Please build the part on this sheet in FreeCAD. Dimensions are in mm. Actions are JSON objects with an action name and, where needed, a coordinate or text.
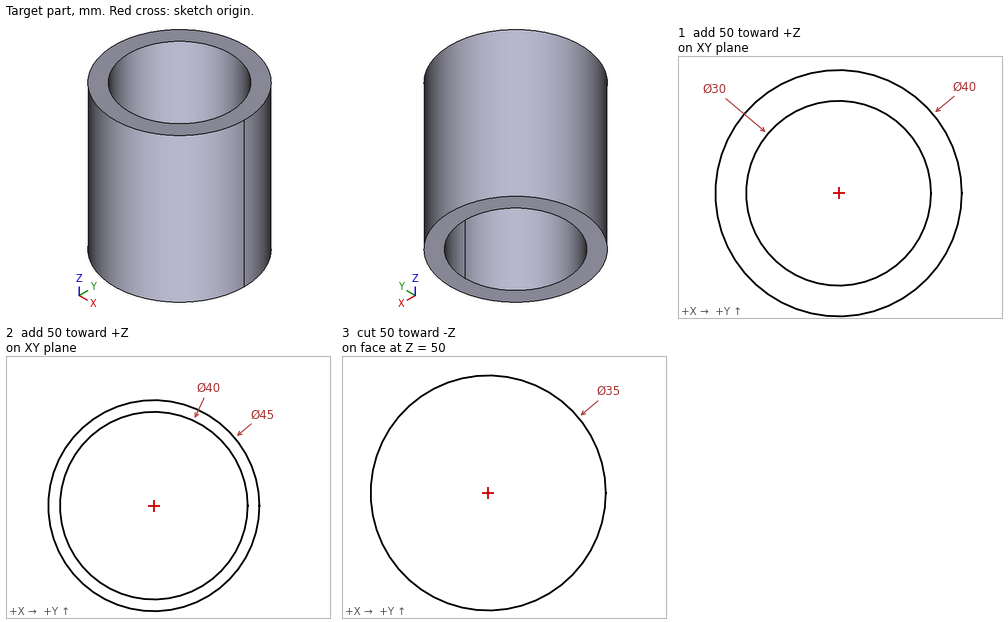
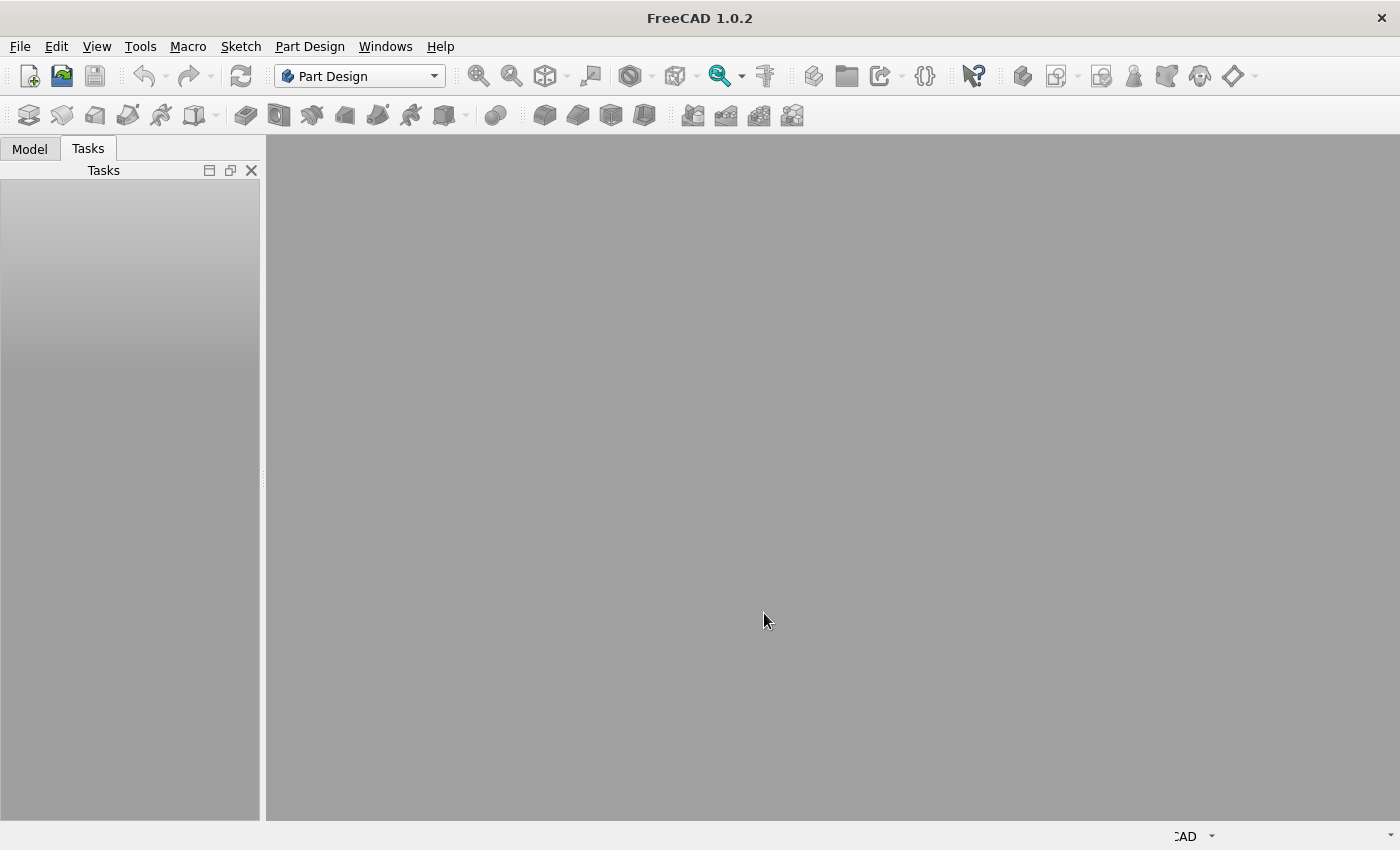
{"action": "left_click", "coordinate": [29, 76]}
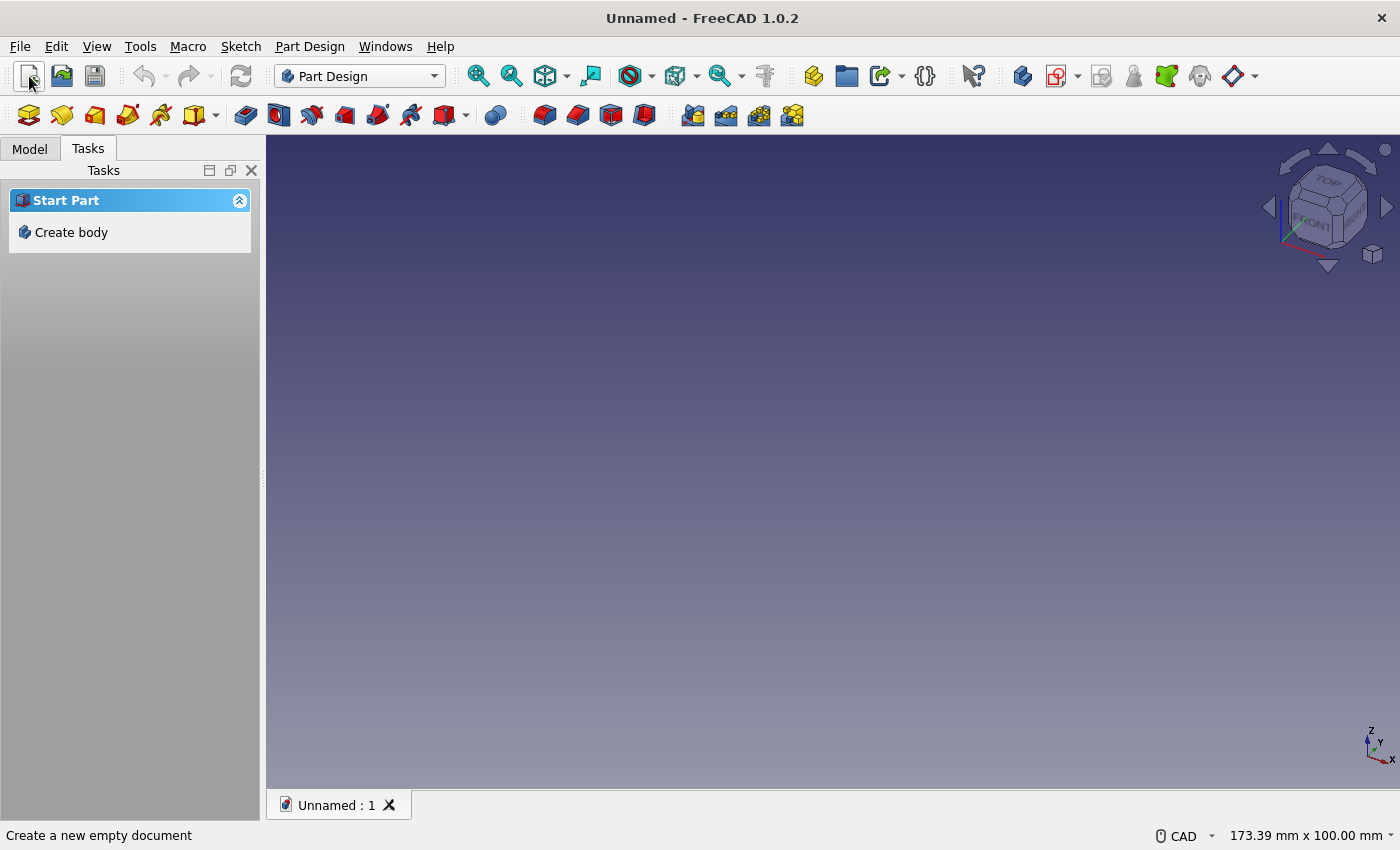
{"action": "left_click", "coordinate": [1056, 76]}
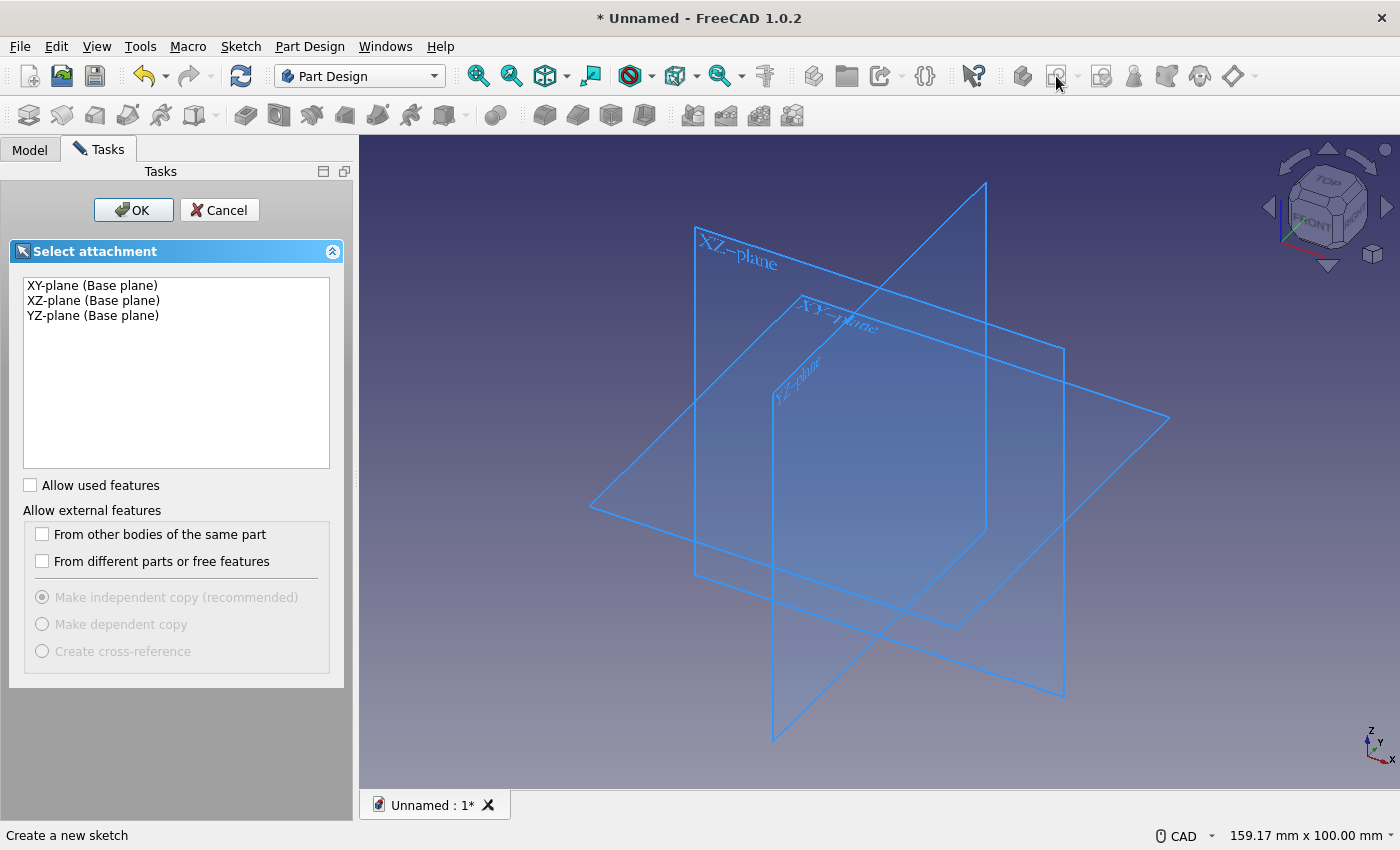
{"action": "left_click", "coordinate": [84, 286]}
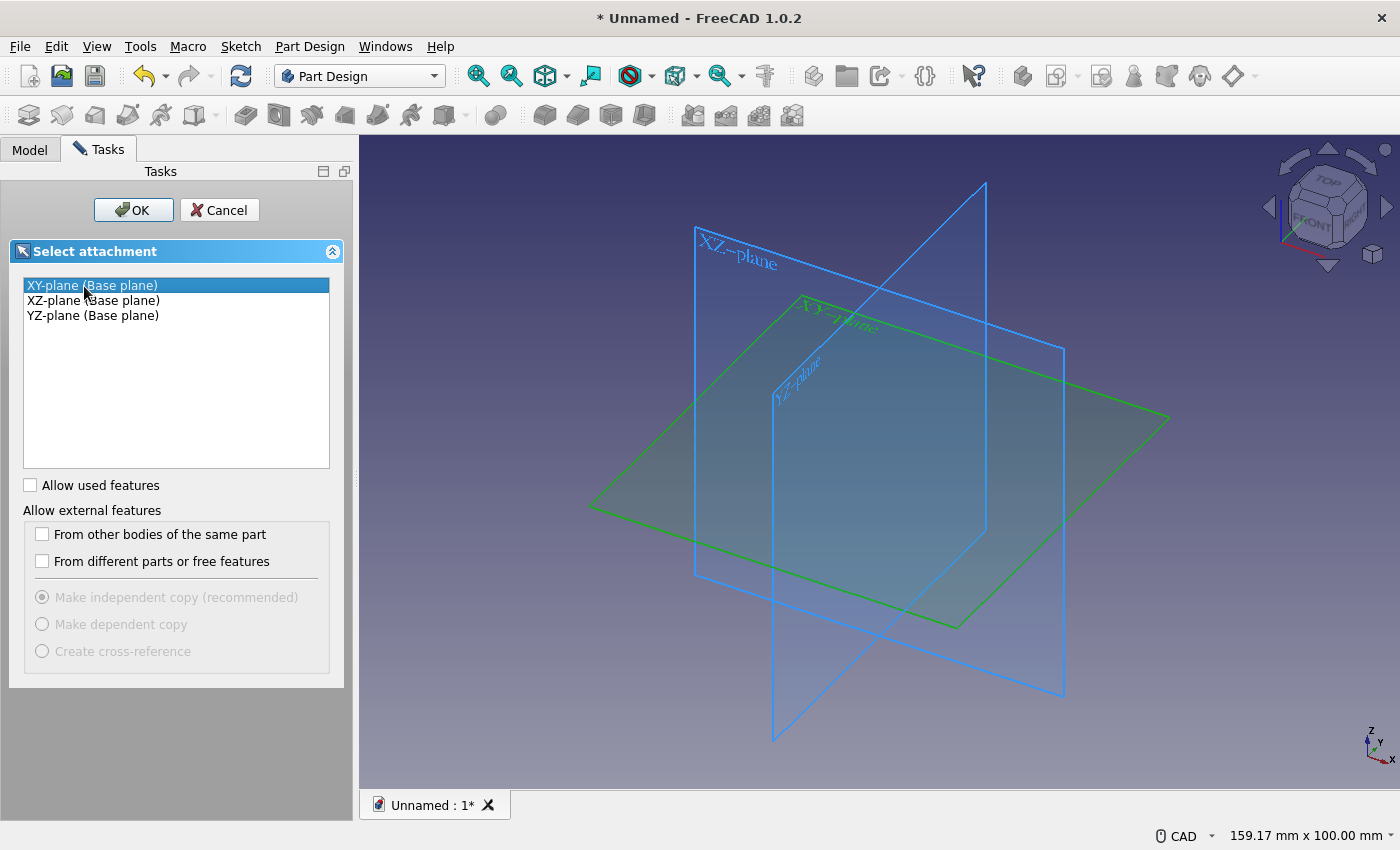
{"action": "left_click", "coordinate": [134, 210]}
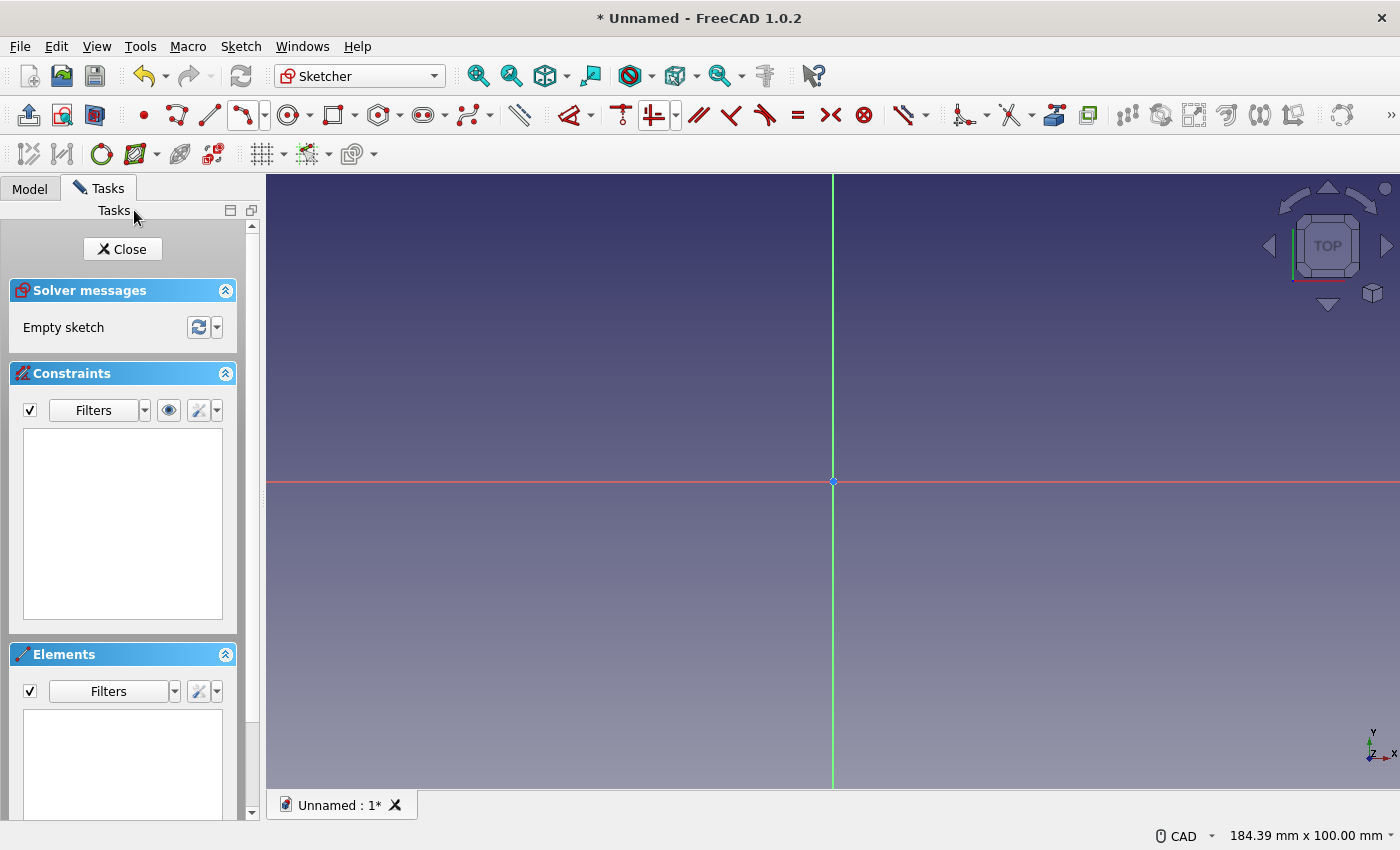
{"action": "scroll", "coordinate": [972, 482], "scroll_direction": "up", "scroll_amount": 2}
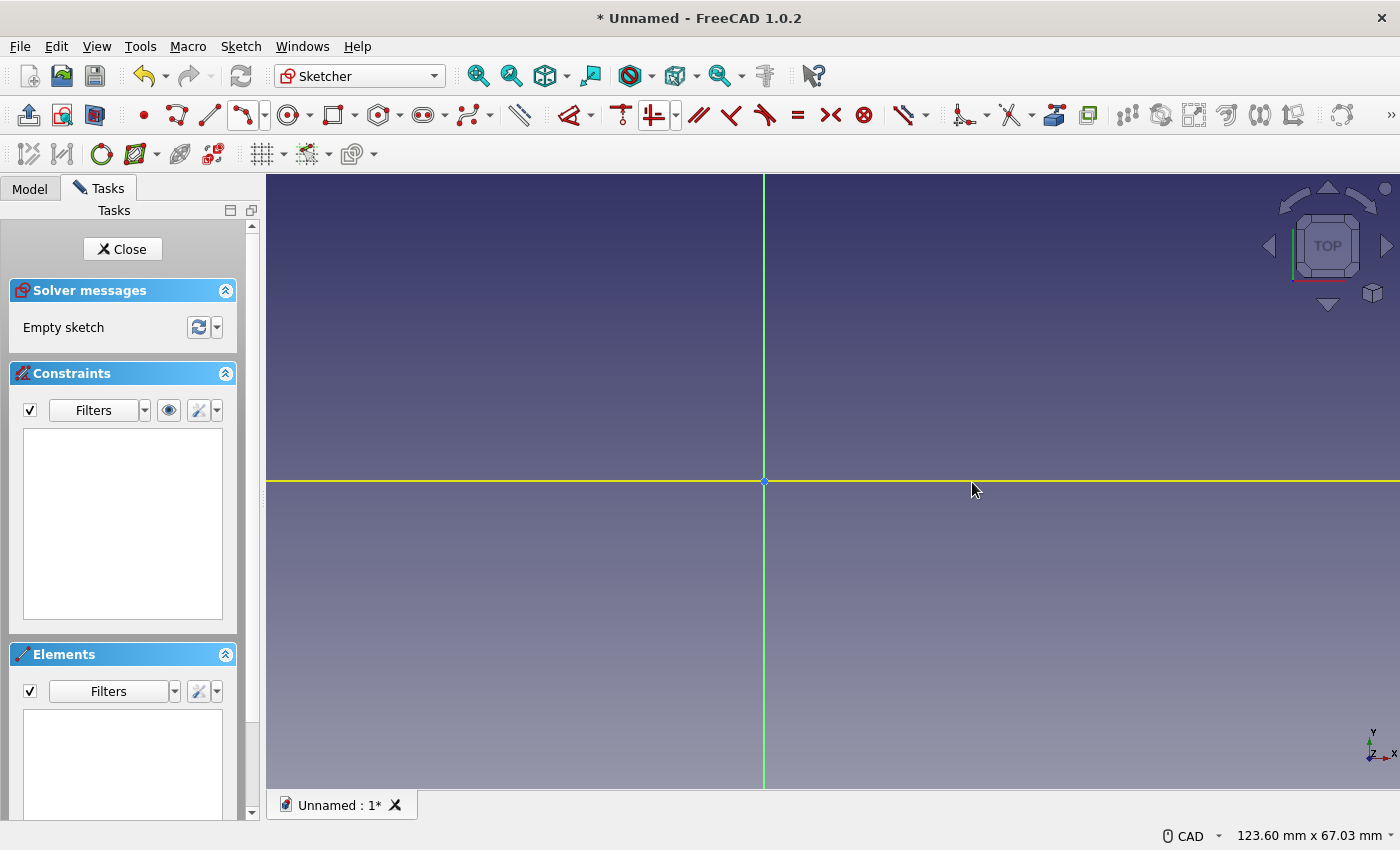
{"action": "key", "text": "g c"}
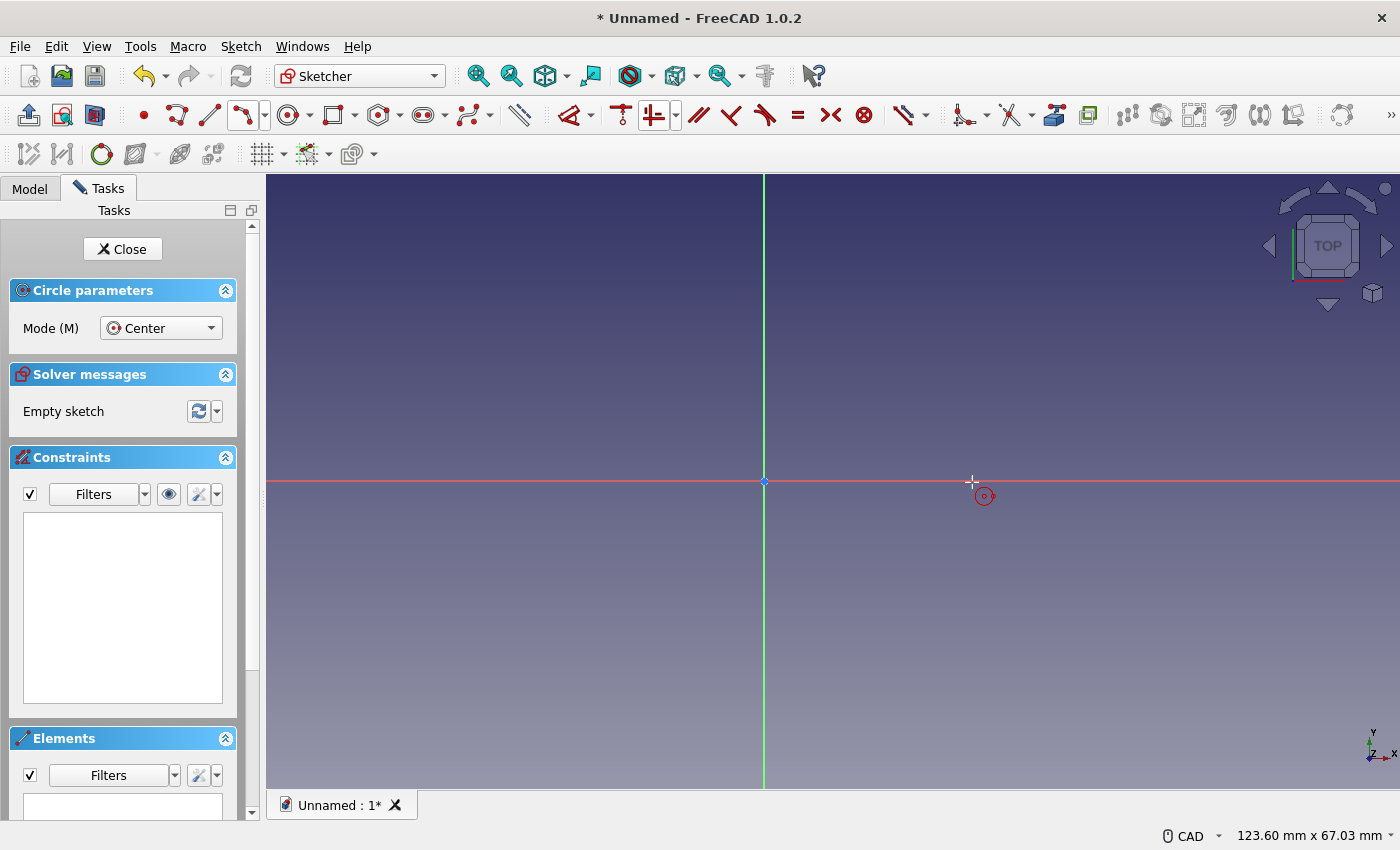
{"action": "left_click", "coordinate": [764, 481]}
{"action": "mouse_move", "coordinate": [894, 351]}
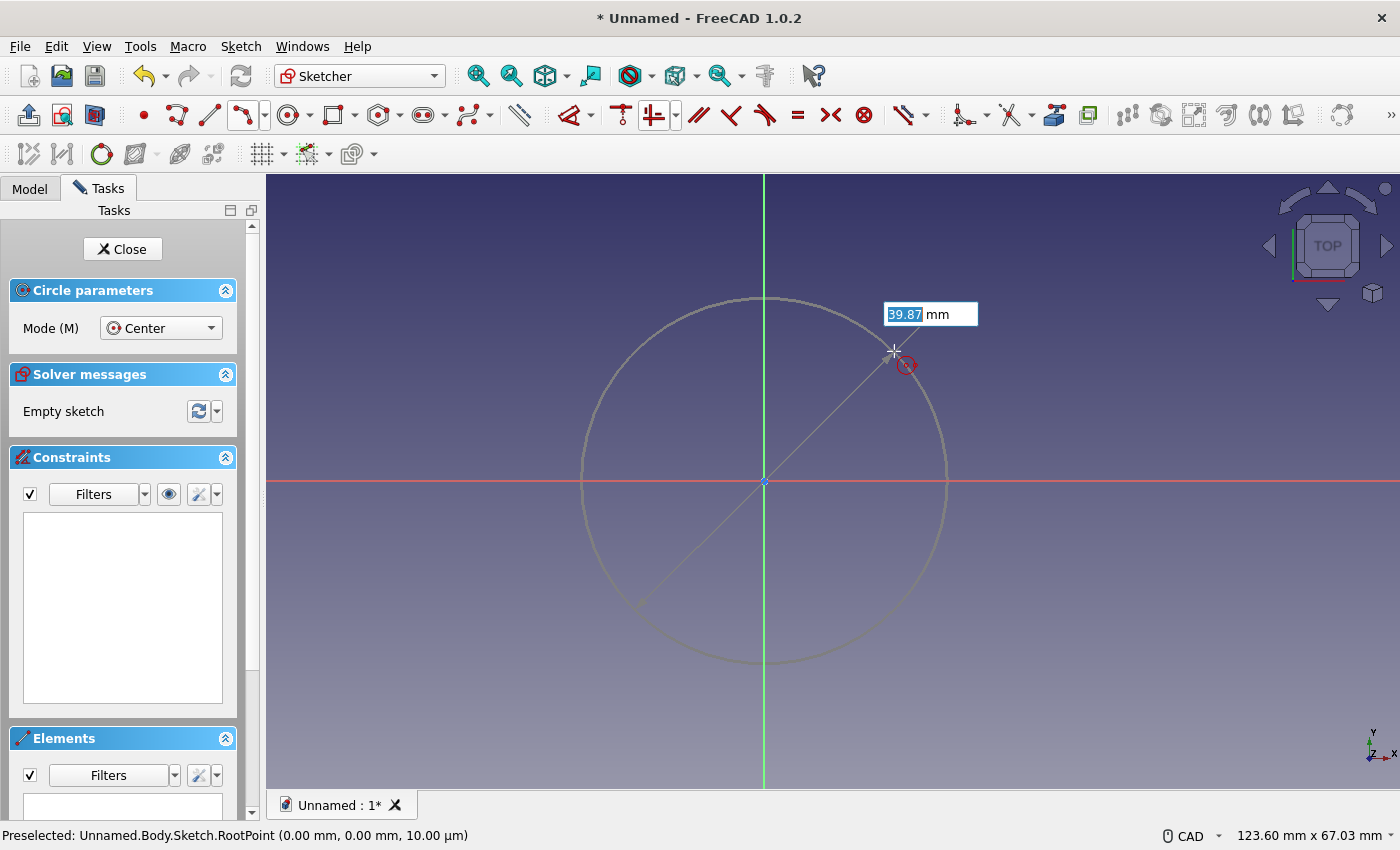
{"action": "type", "text": "40"}
{"action": "key", "text": "Return"}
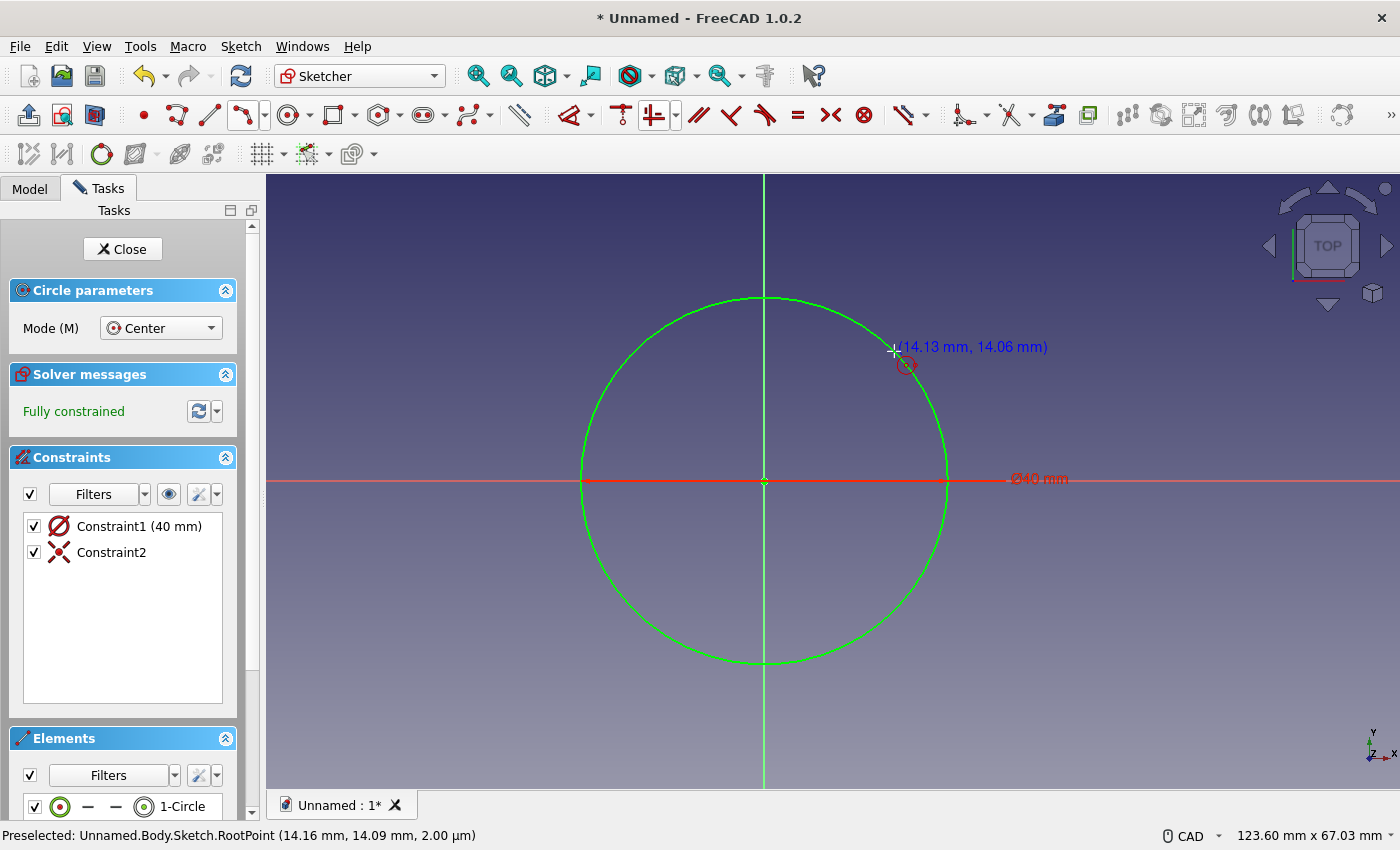
{"action": "left_click", "coordinate": [764, 481]}
{"action": "mouse_move", "coordinate": [862, 384]}